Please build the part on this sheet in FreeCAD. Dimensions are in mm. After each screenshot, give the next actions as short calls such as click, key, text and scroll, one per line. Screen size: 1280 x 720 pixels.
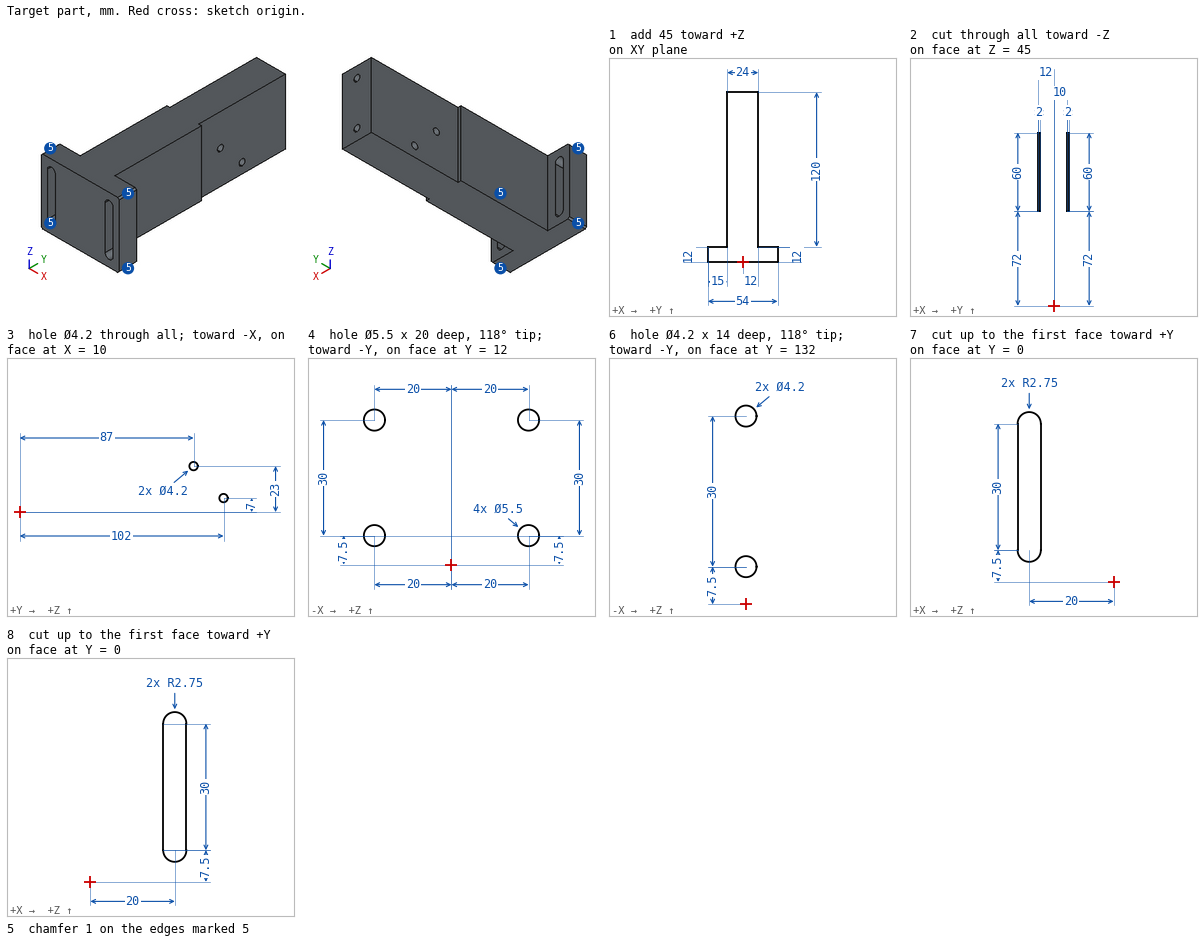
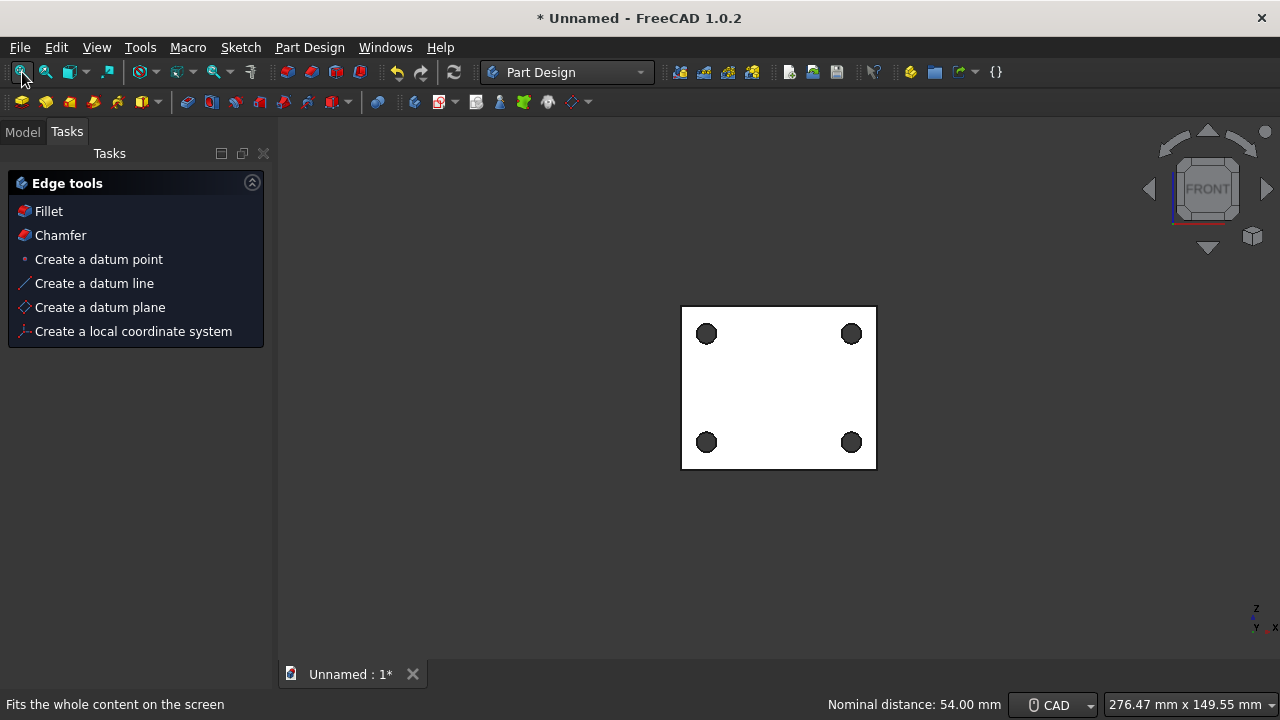
key(3)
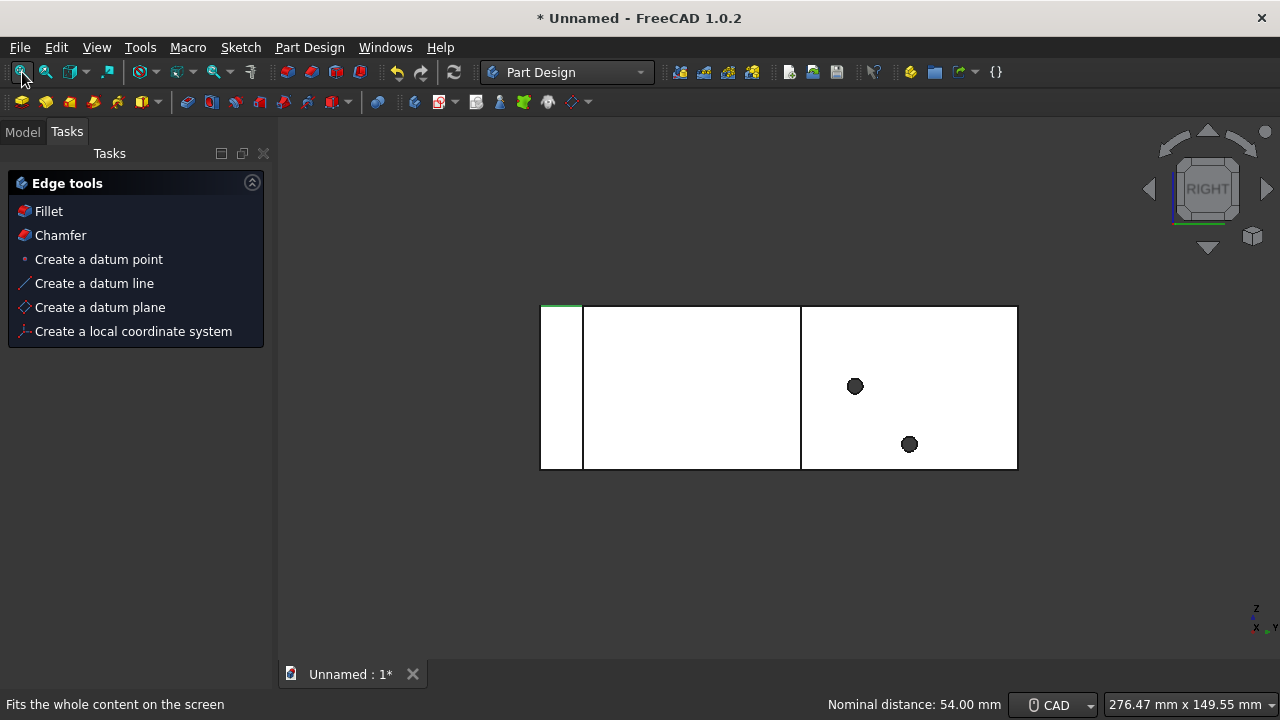
click(562, 469, ctrl)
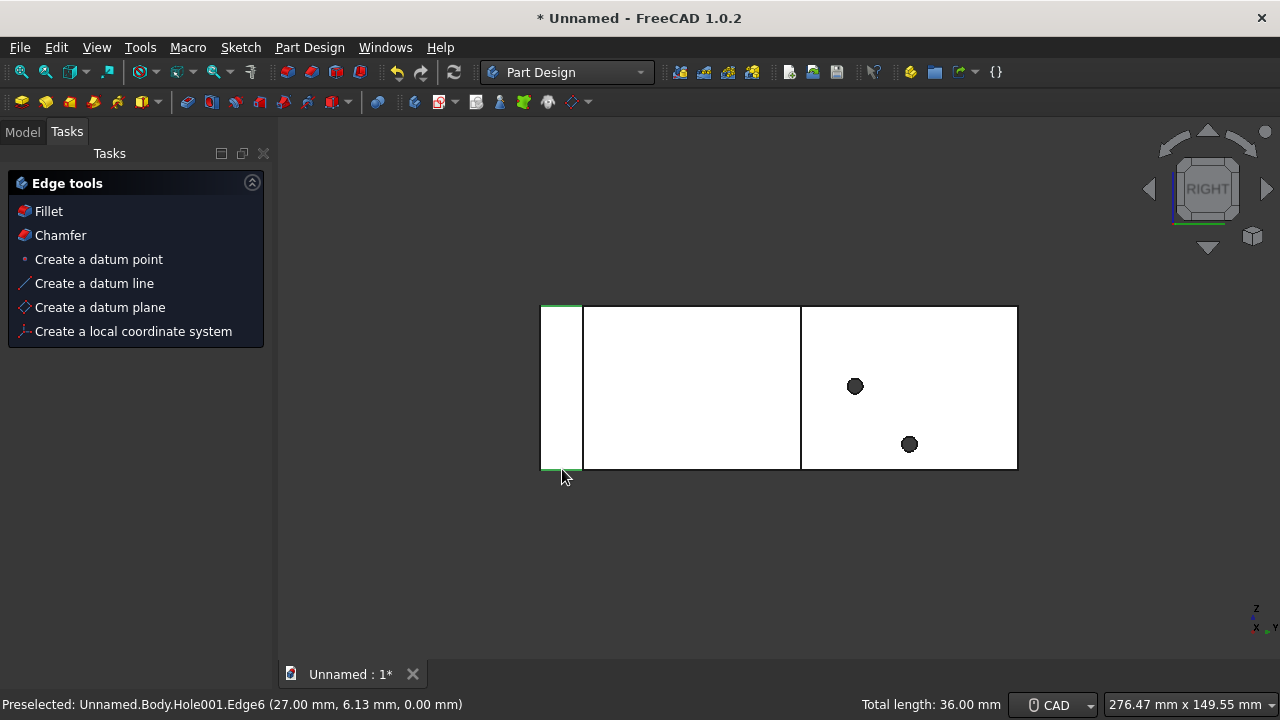
key(5)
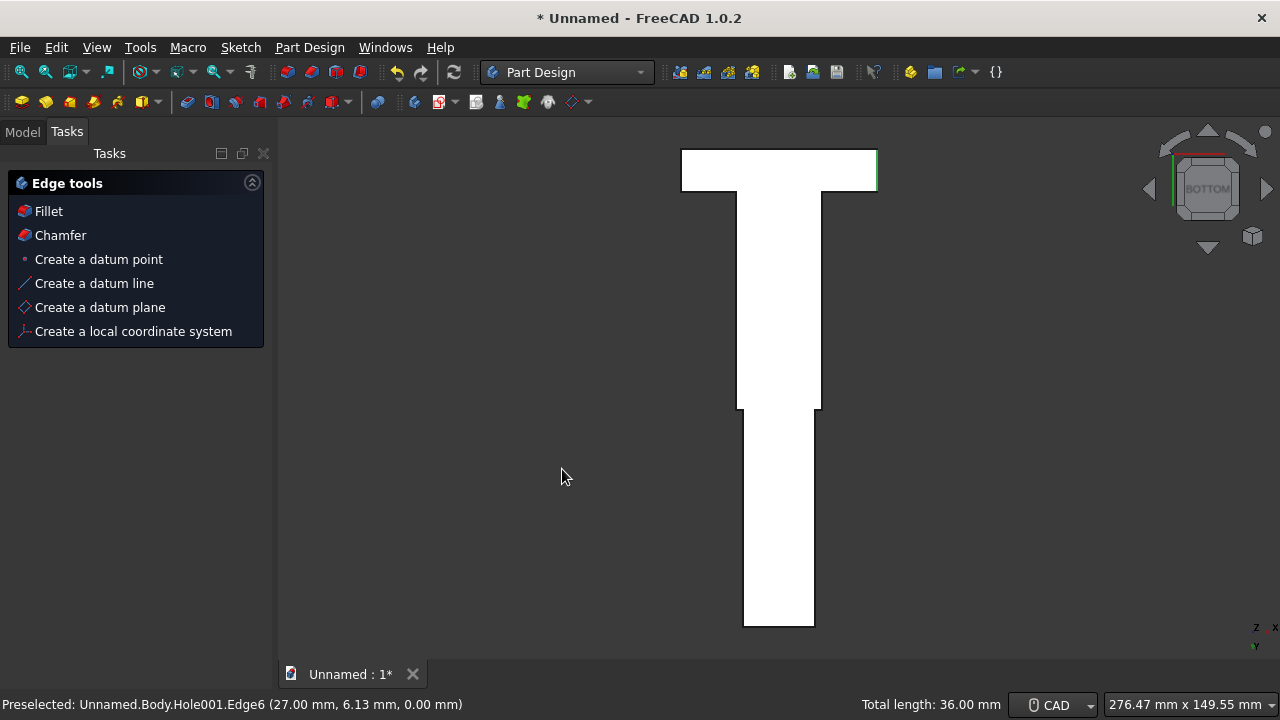
click(681, 170, ctrl)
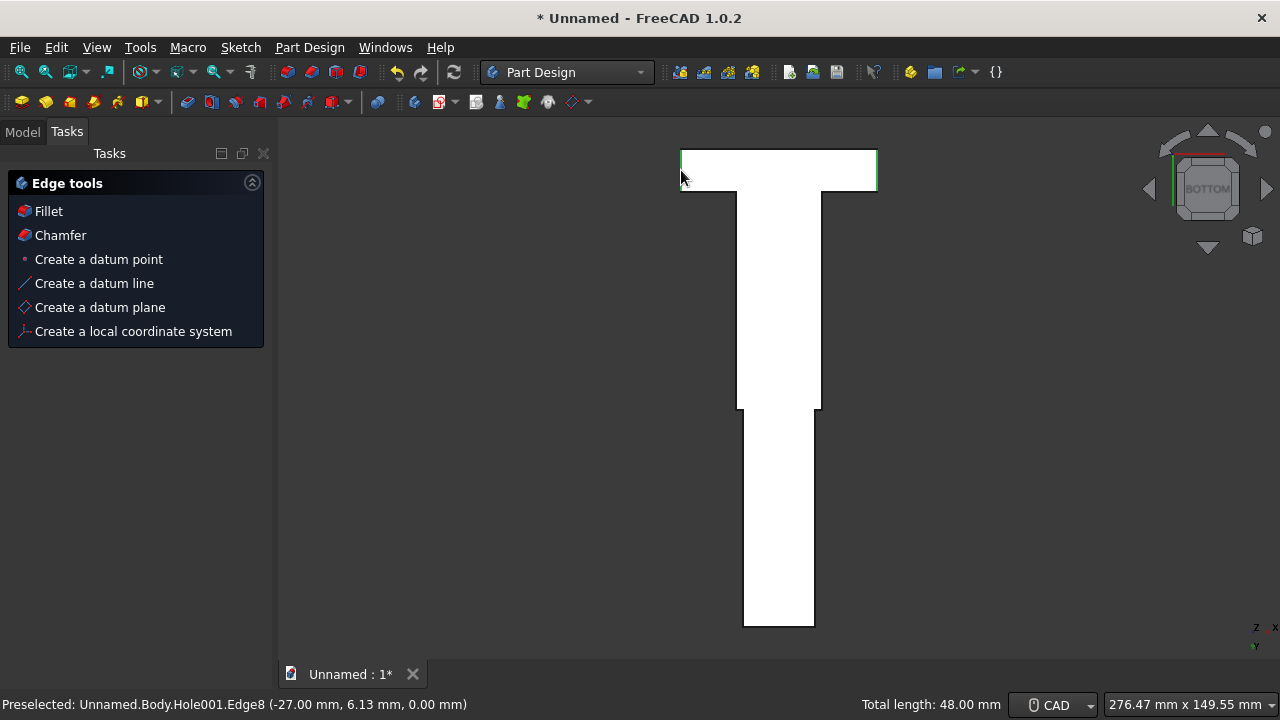
click(312, 72)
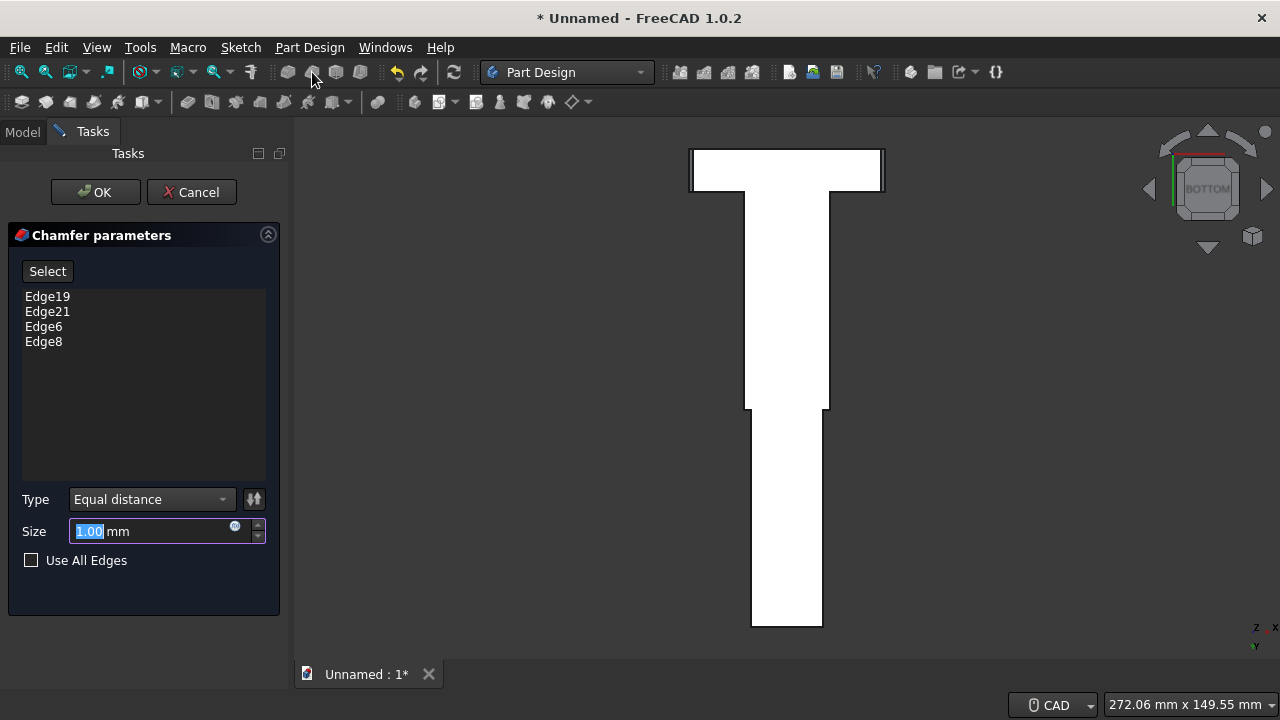
text(1)
key(Tab)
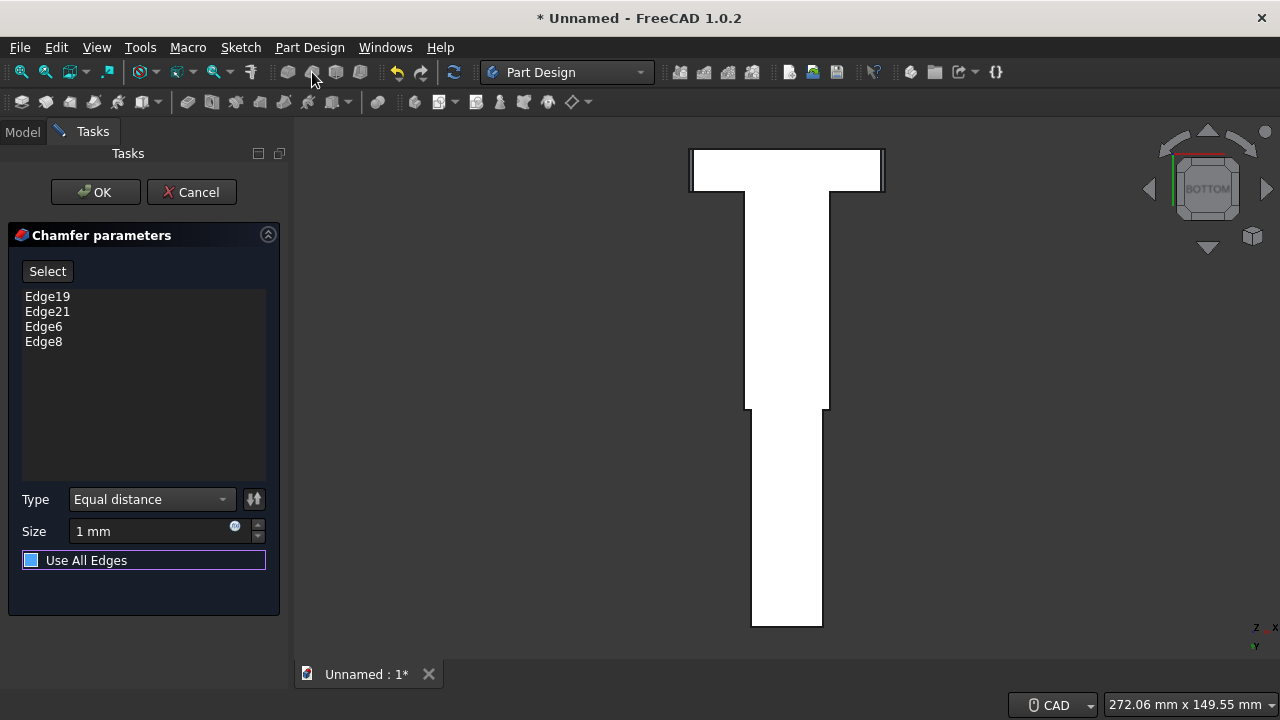
click(96, 192)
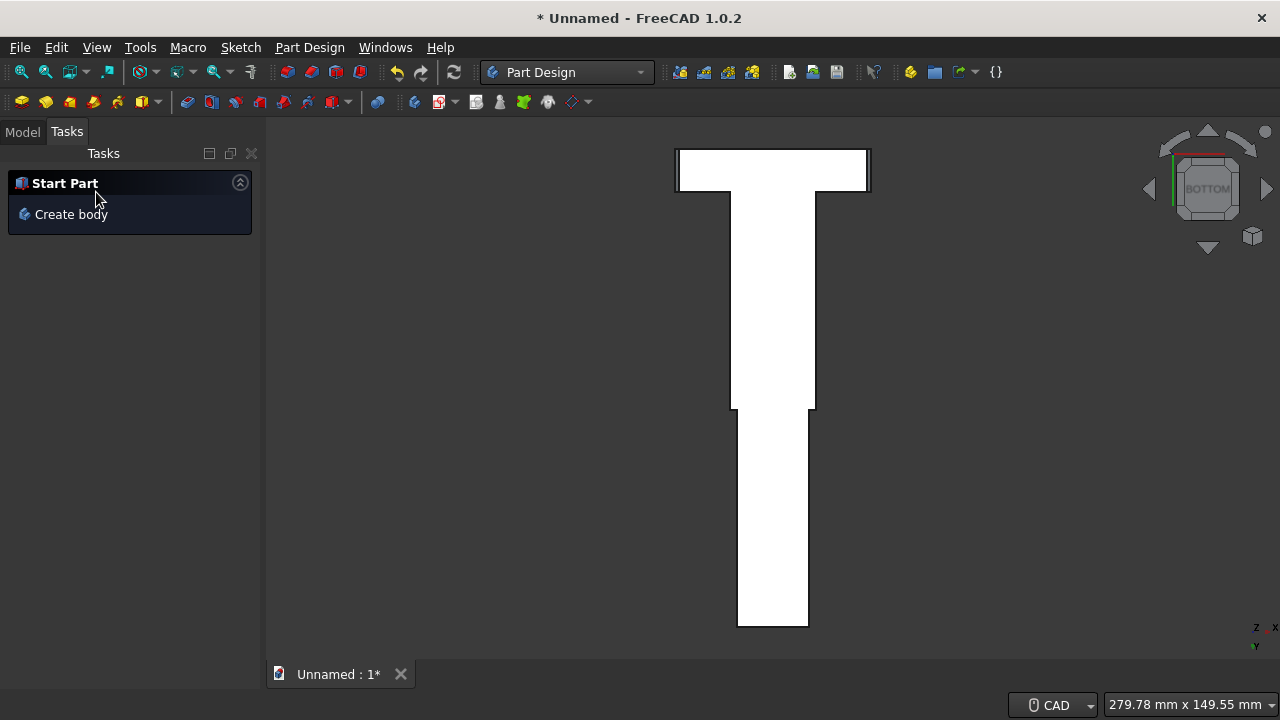
key(4)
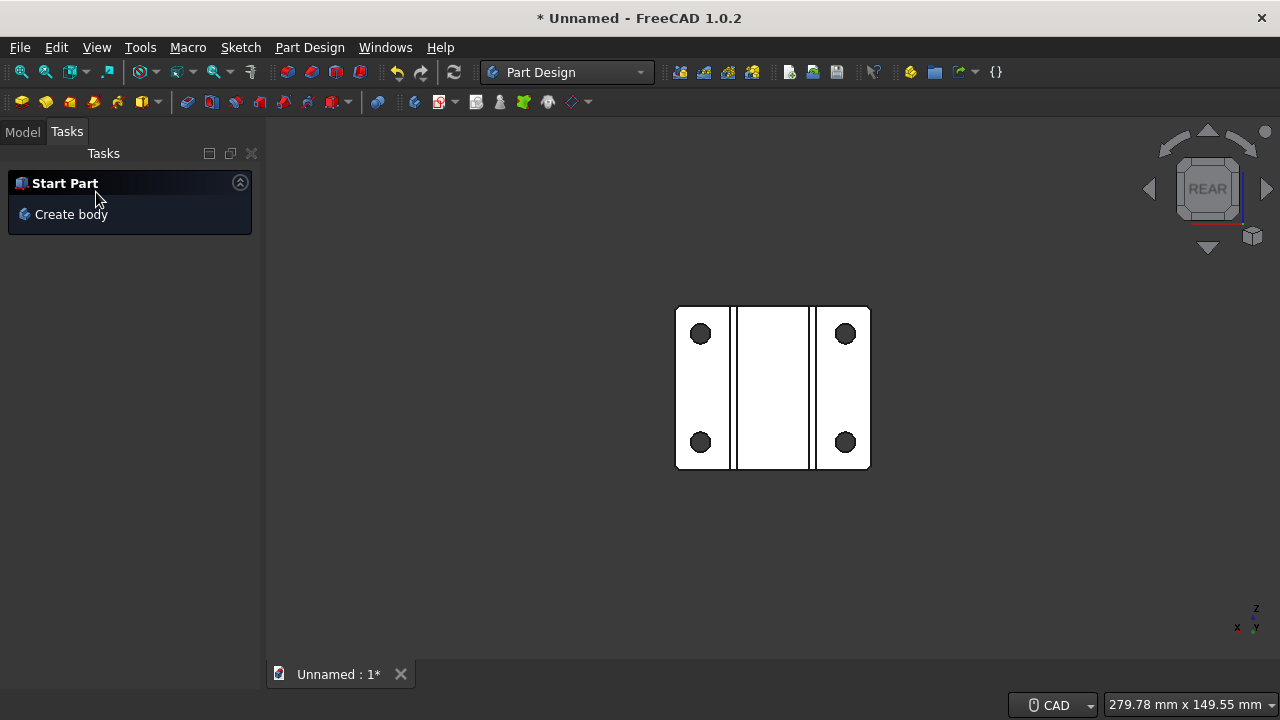
click(22, 72)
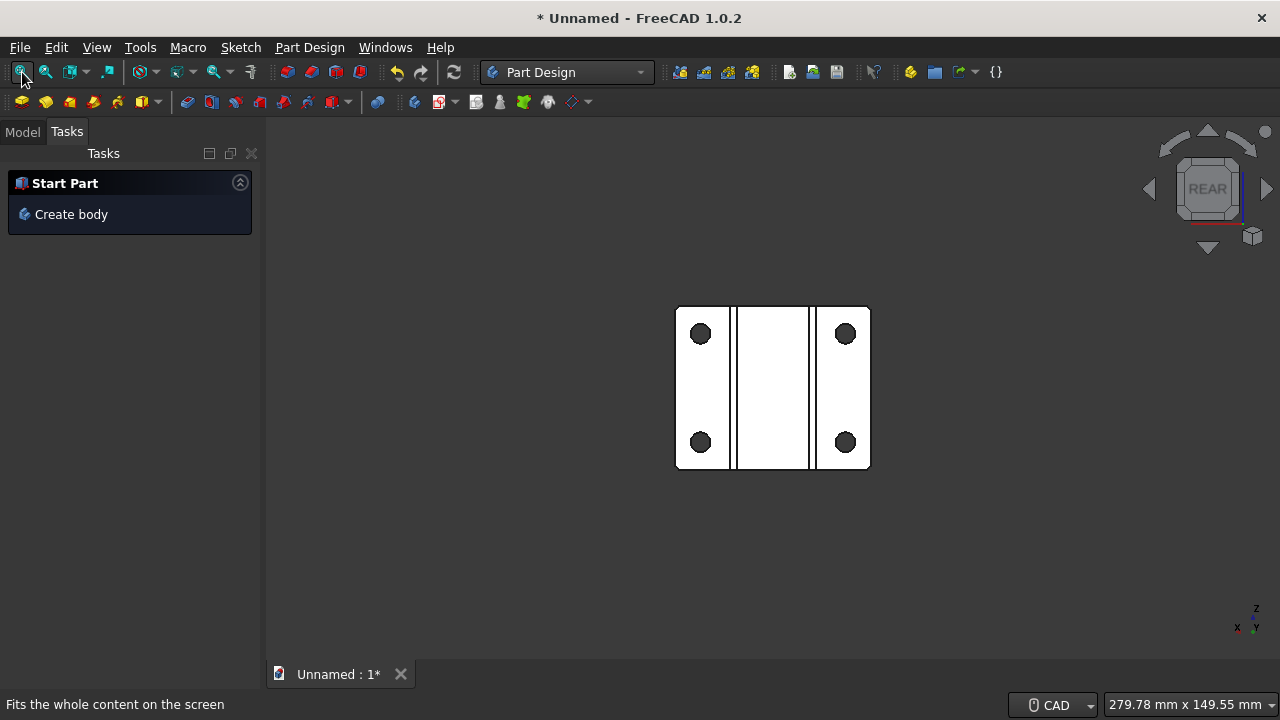
click(773, 364)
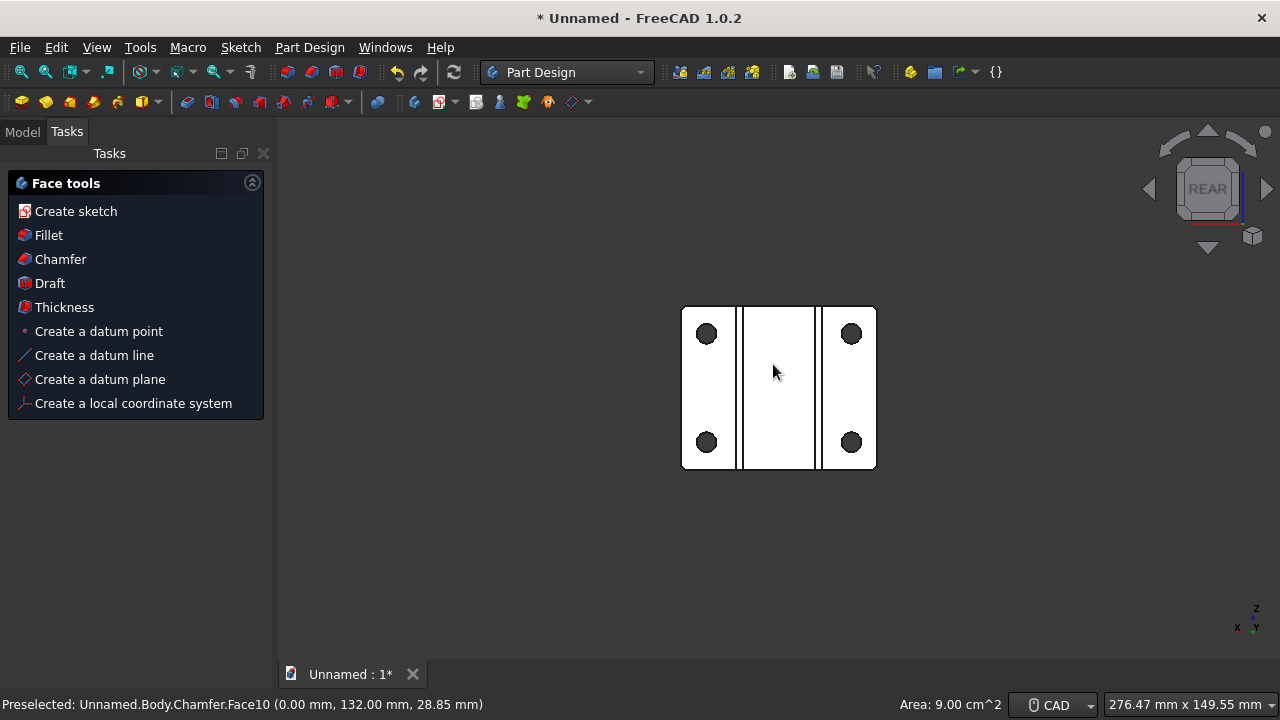
click(440, 102)